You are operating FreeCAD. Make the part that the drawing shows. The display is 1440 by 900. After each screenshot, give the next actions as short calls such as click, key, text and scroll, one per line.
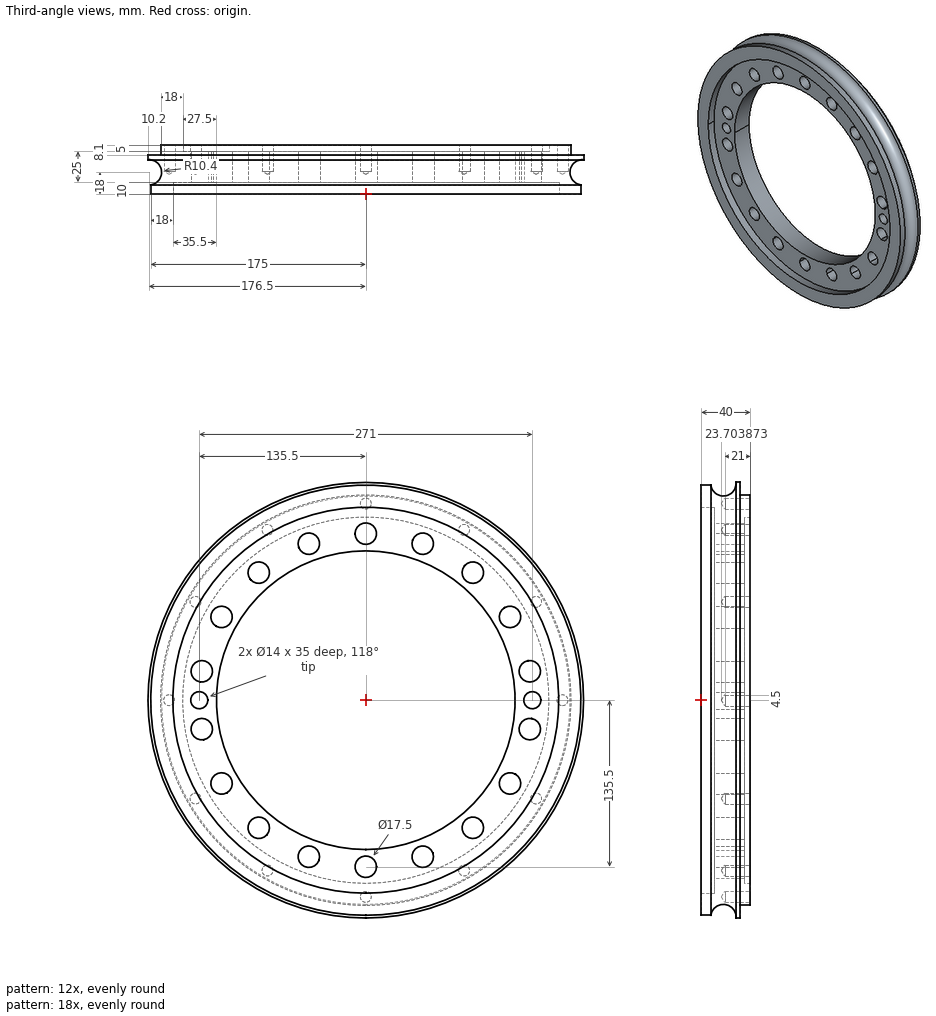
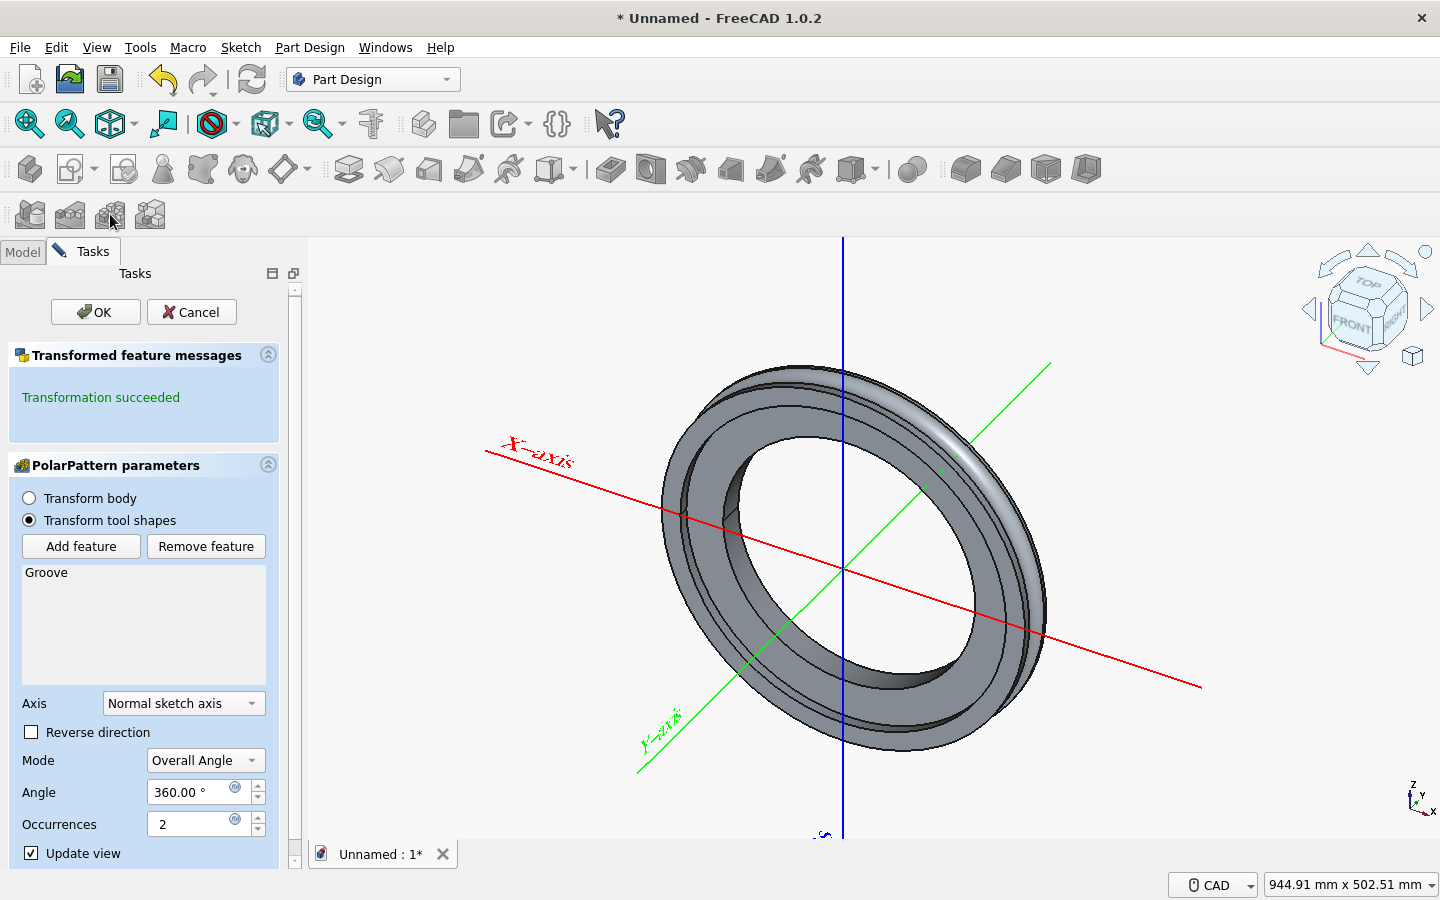
click(184, 704)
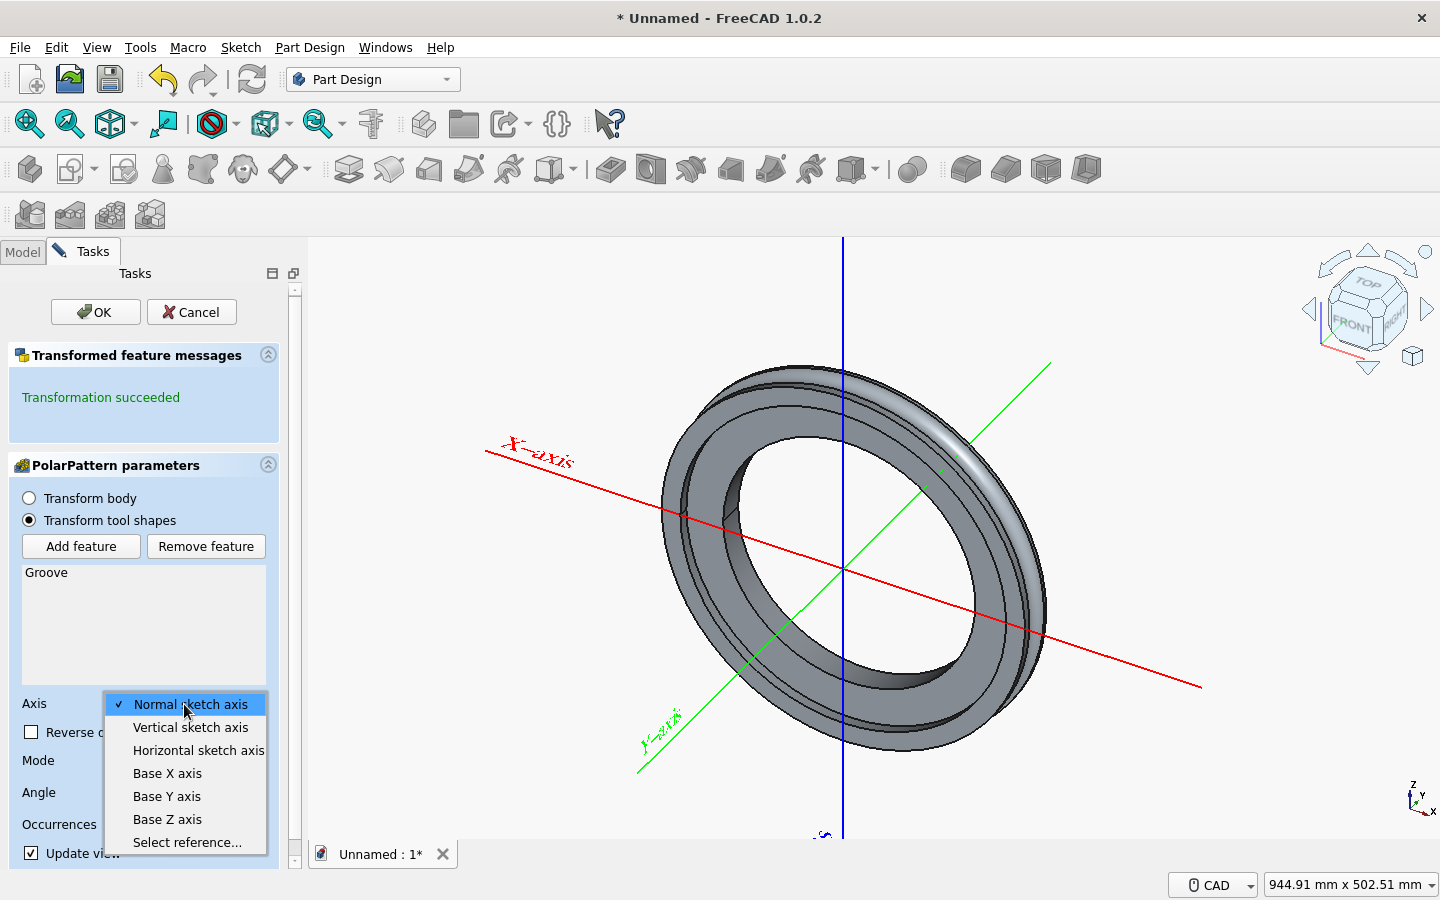
click(184, 796)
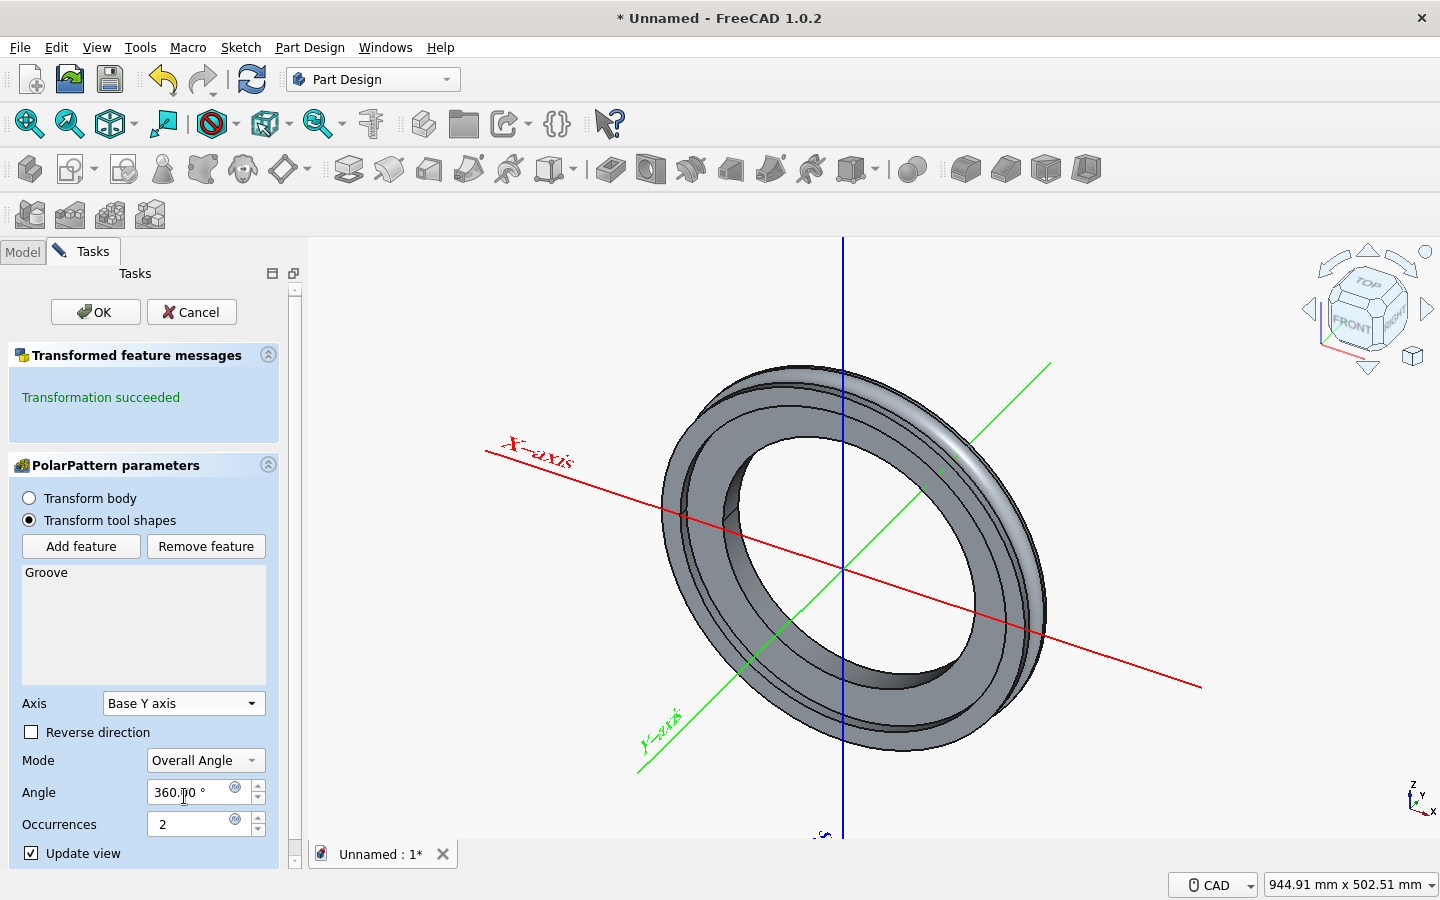
triple_click(198, 824)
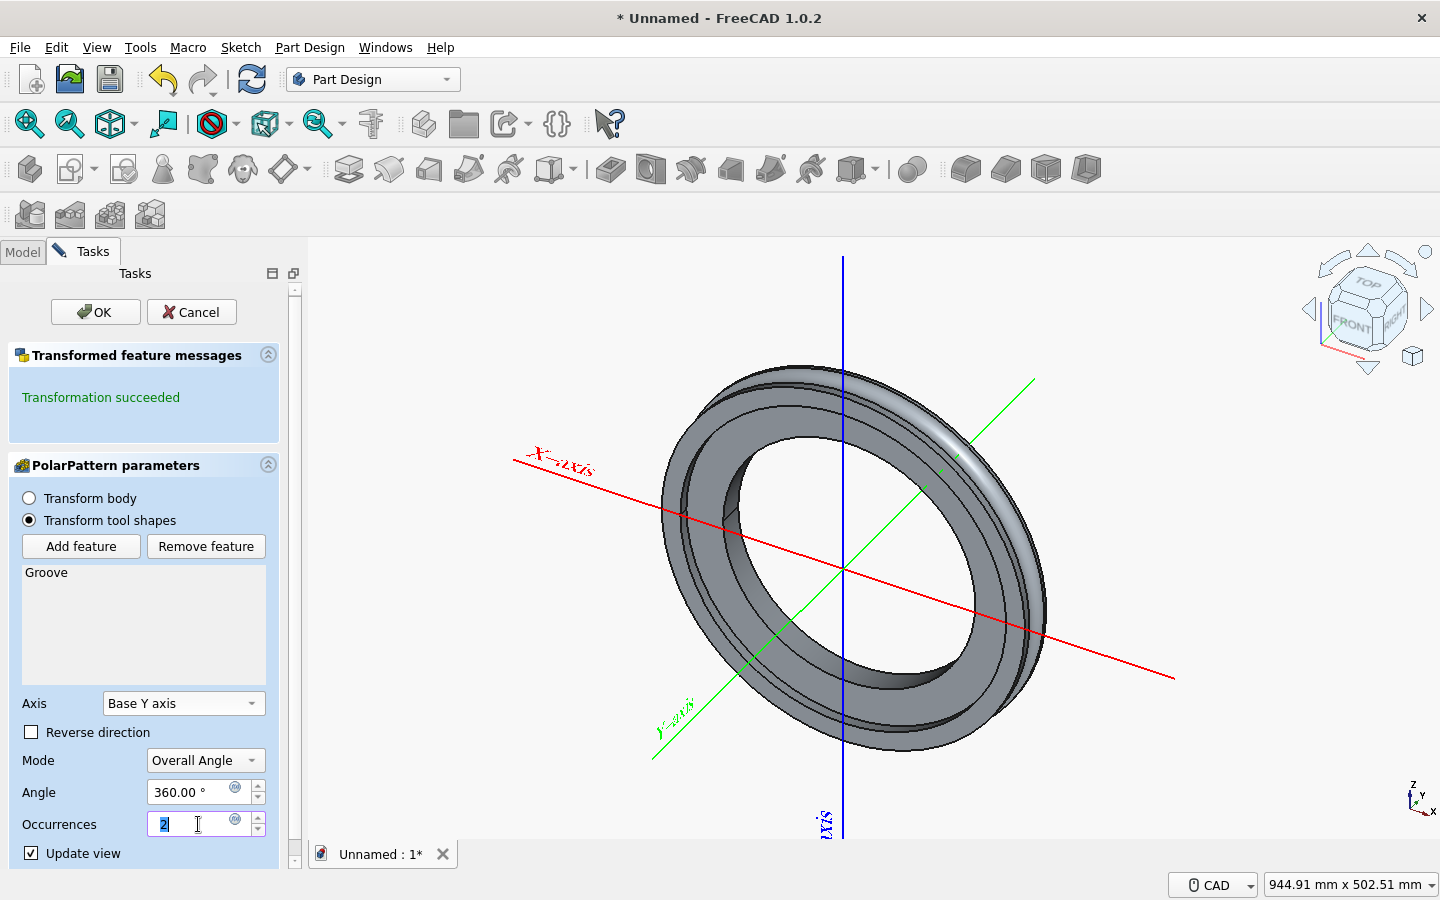
text(12)
key(Tab)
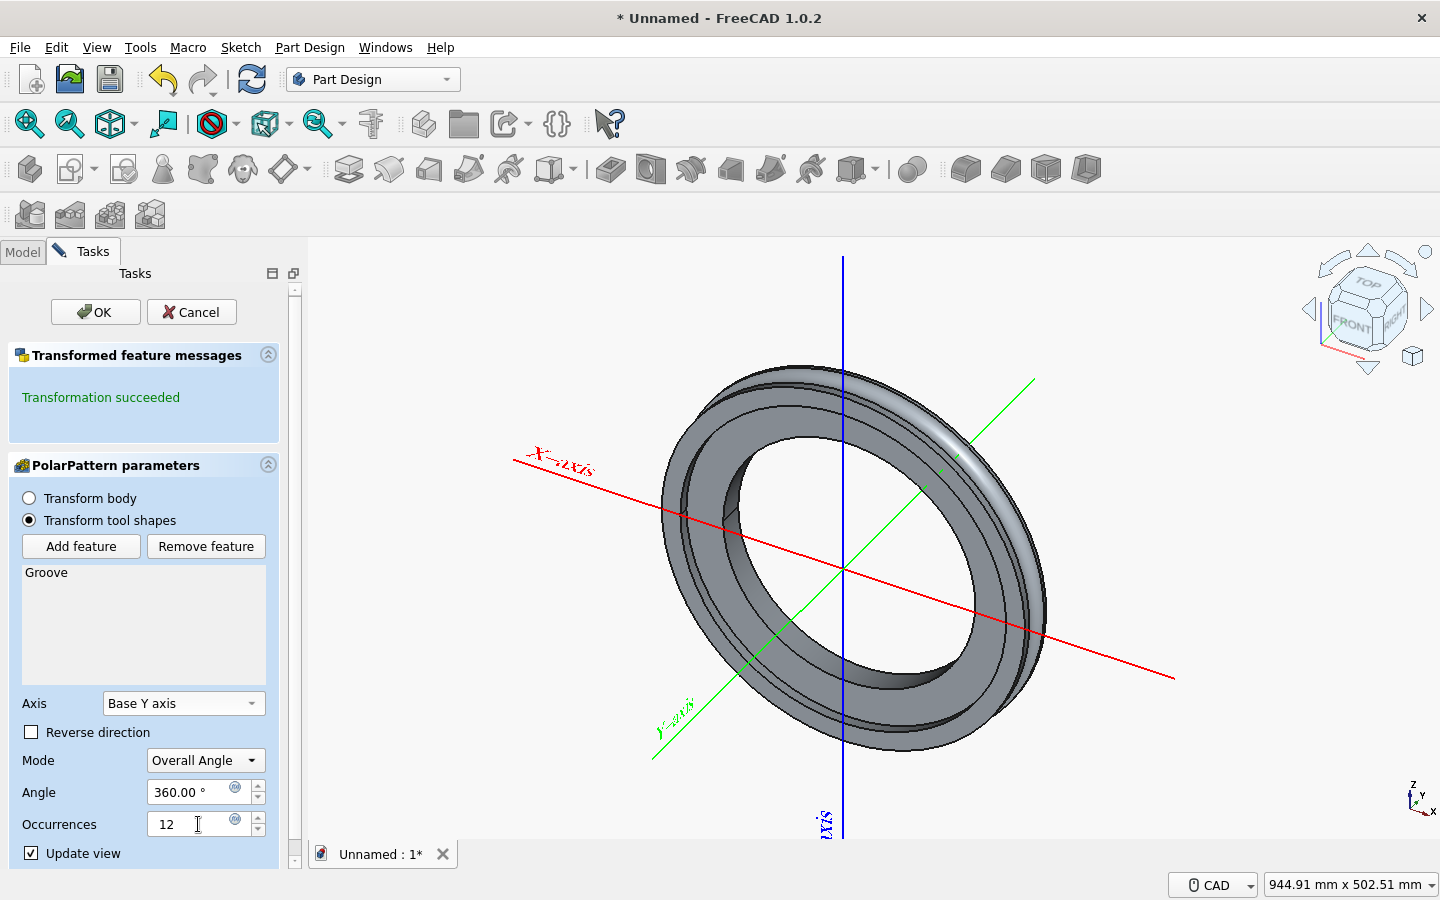
click(96, 312)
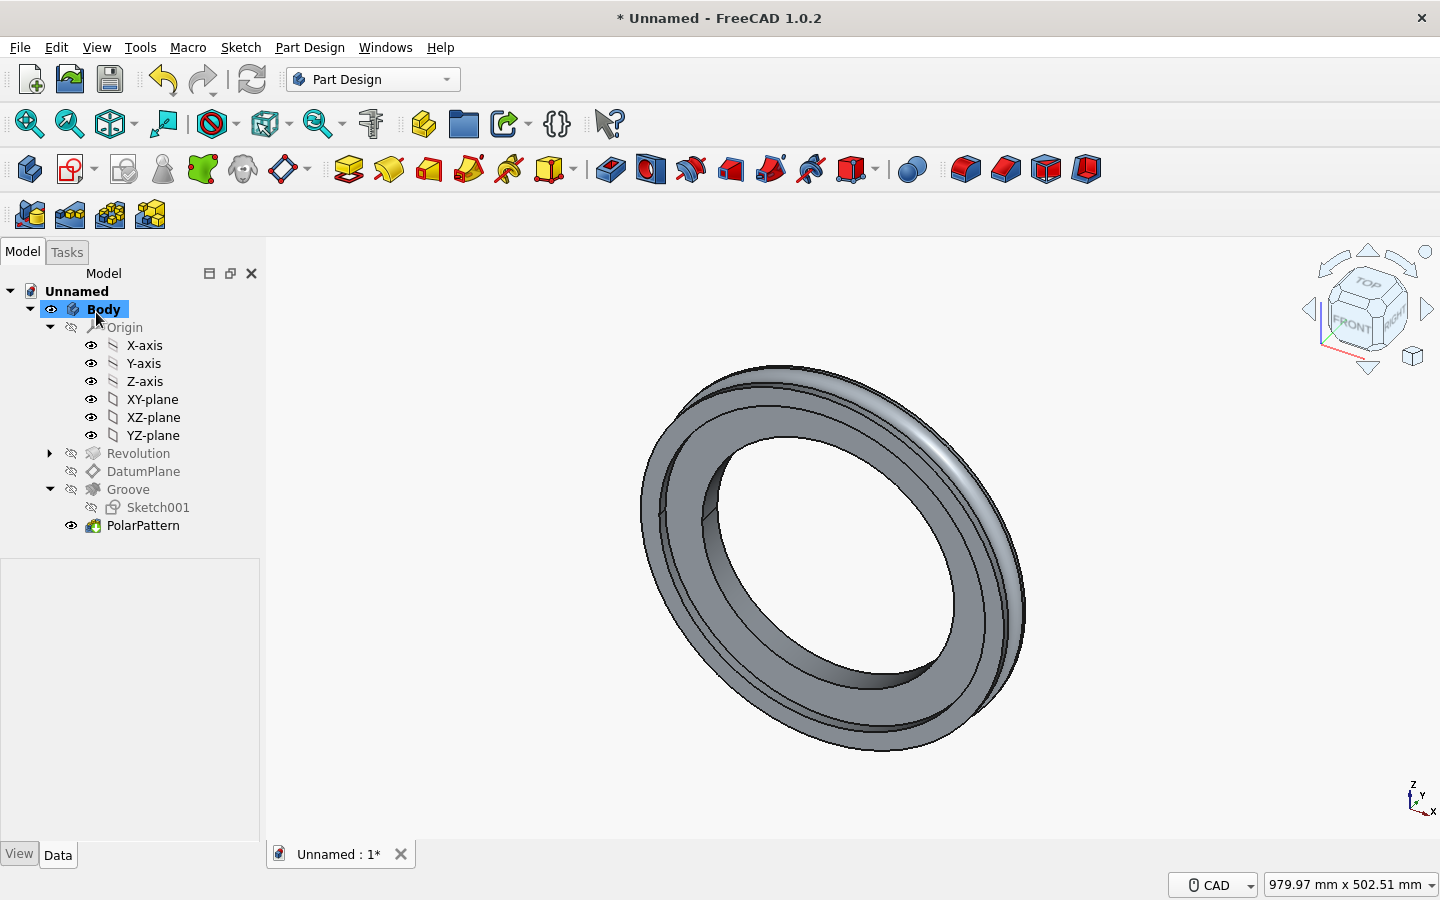
key(4)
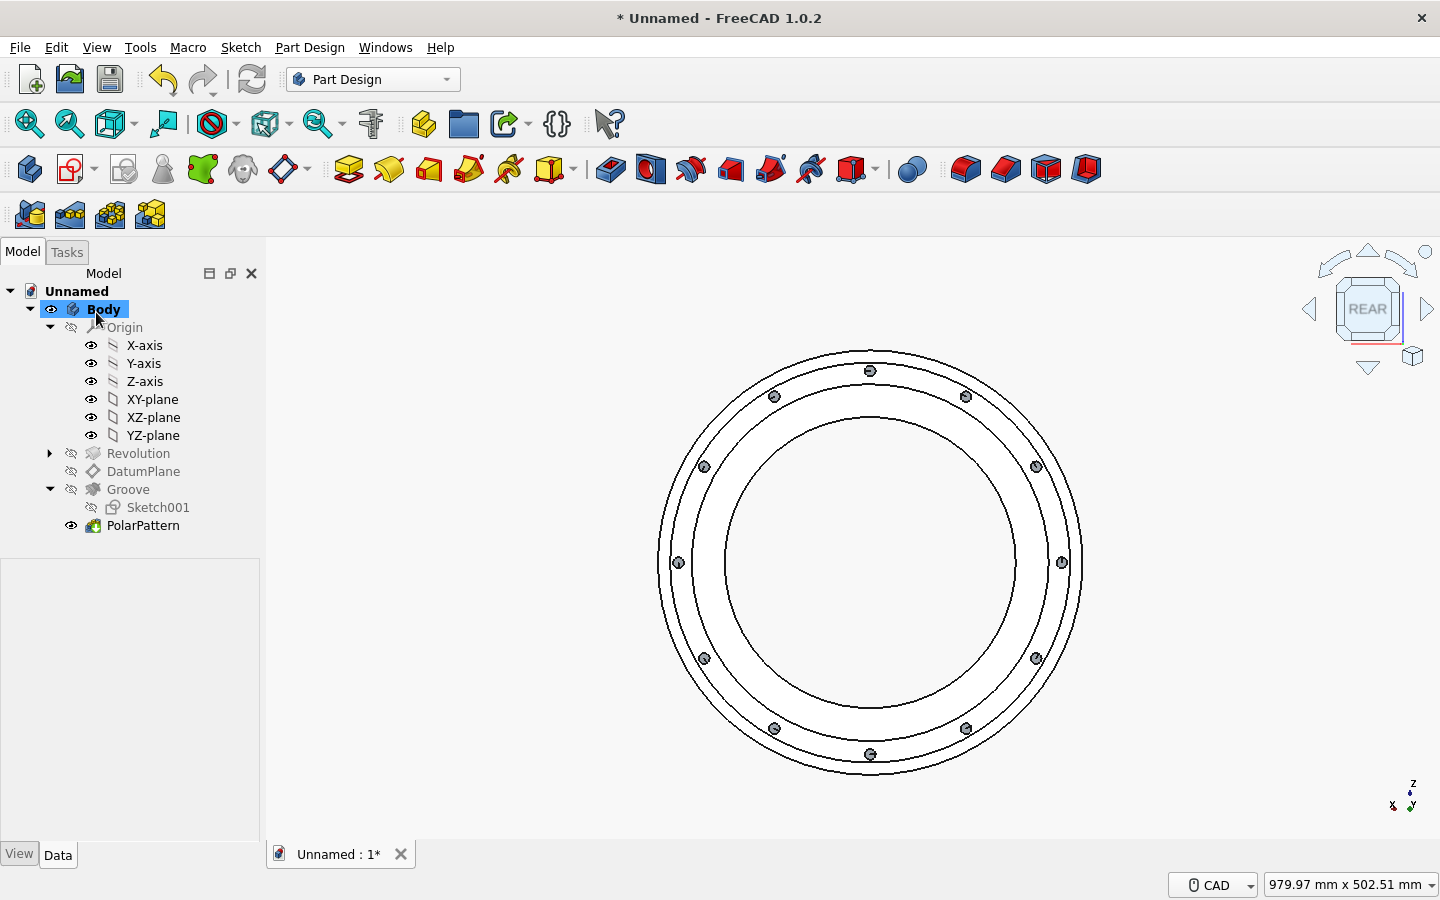
click(717, 511)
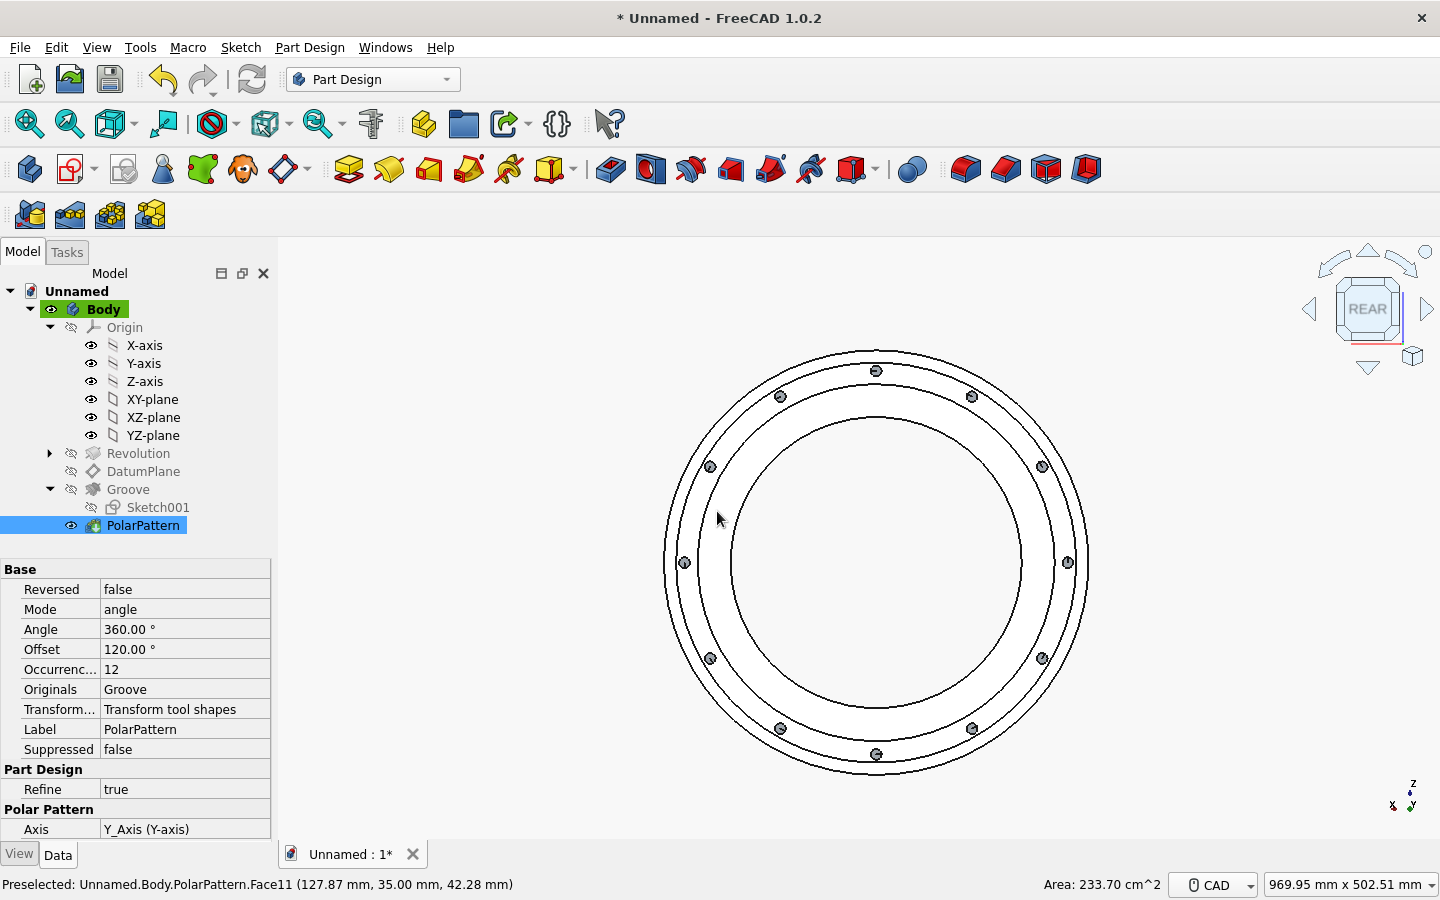
click(70, 170)